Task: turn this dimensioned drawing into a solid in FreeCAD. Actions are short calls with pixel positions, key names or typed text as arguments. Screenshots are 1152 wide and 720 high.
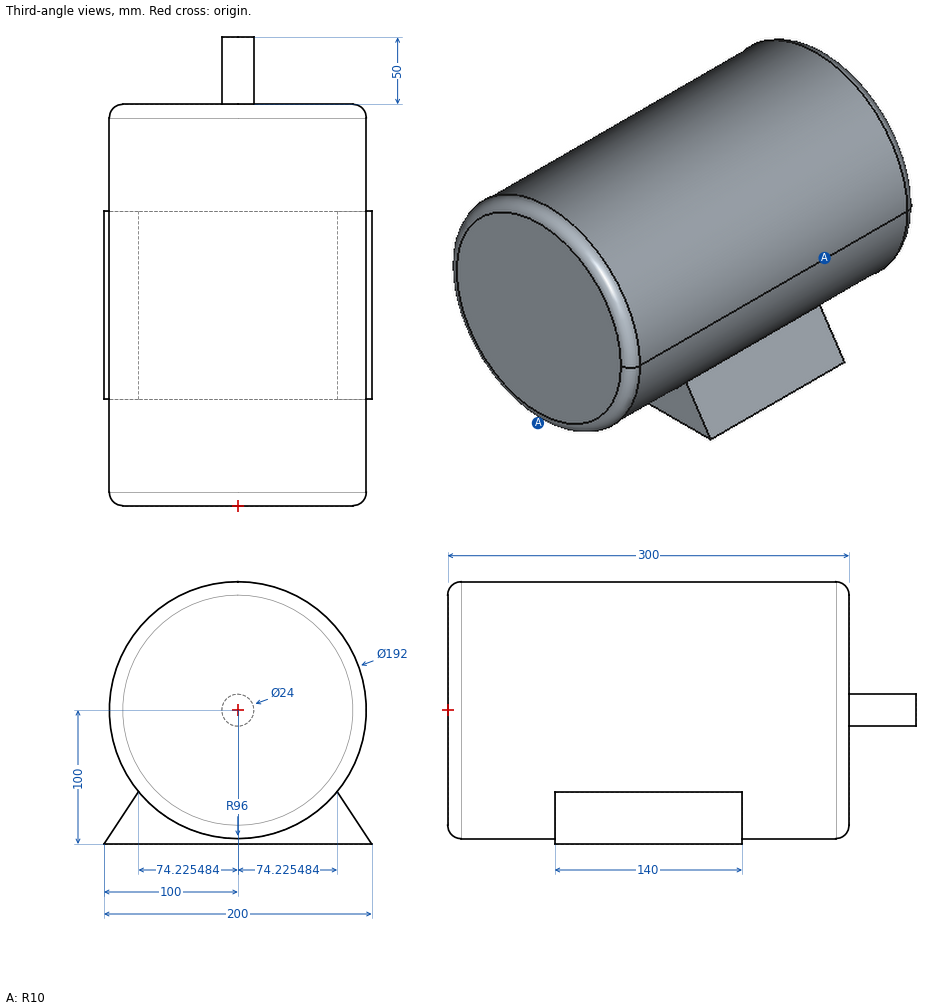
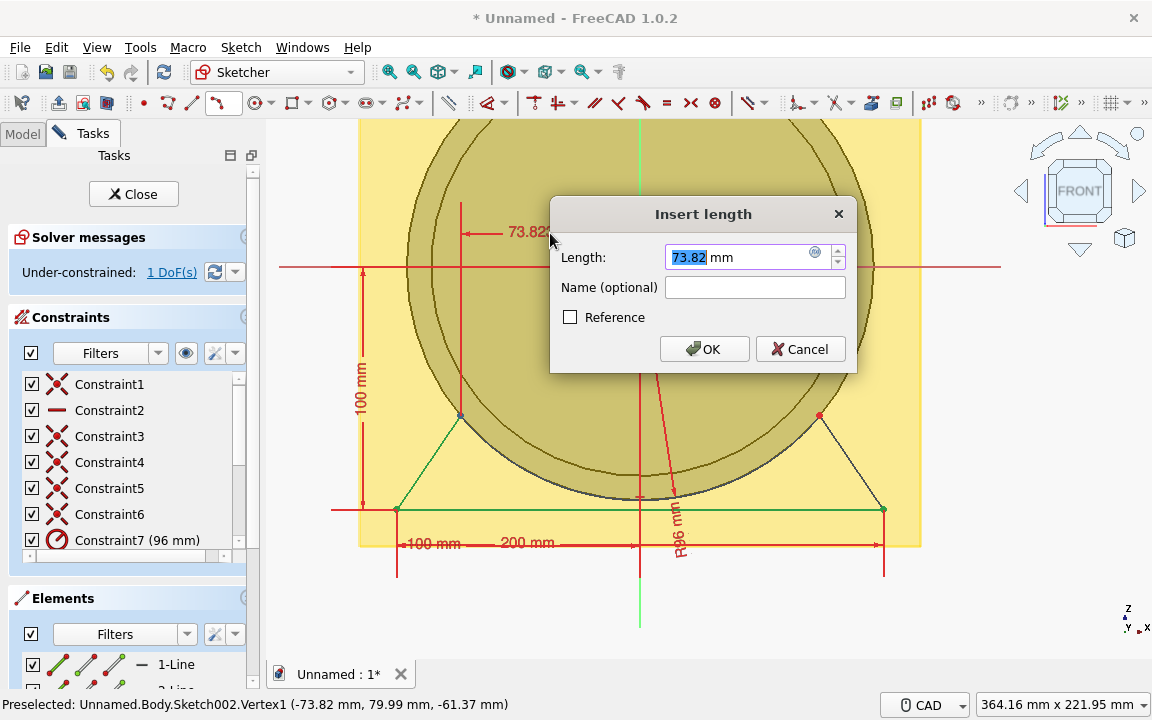
text(74.225484)
key(Return)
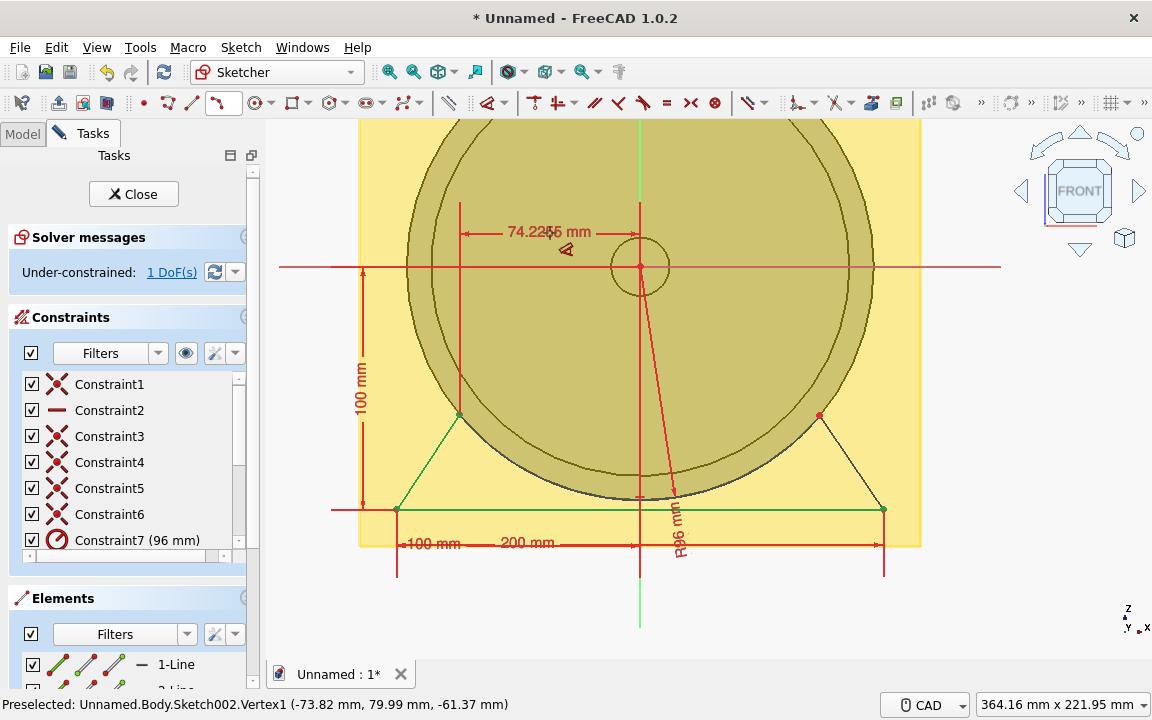
click(820, 416)
click(730, 233)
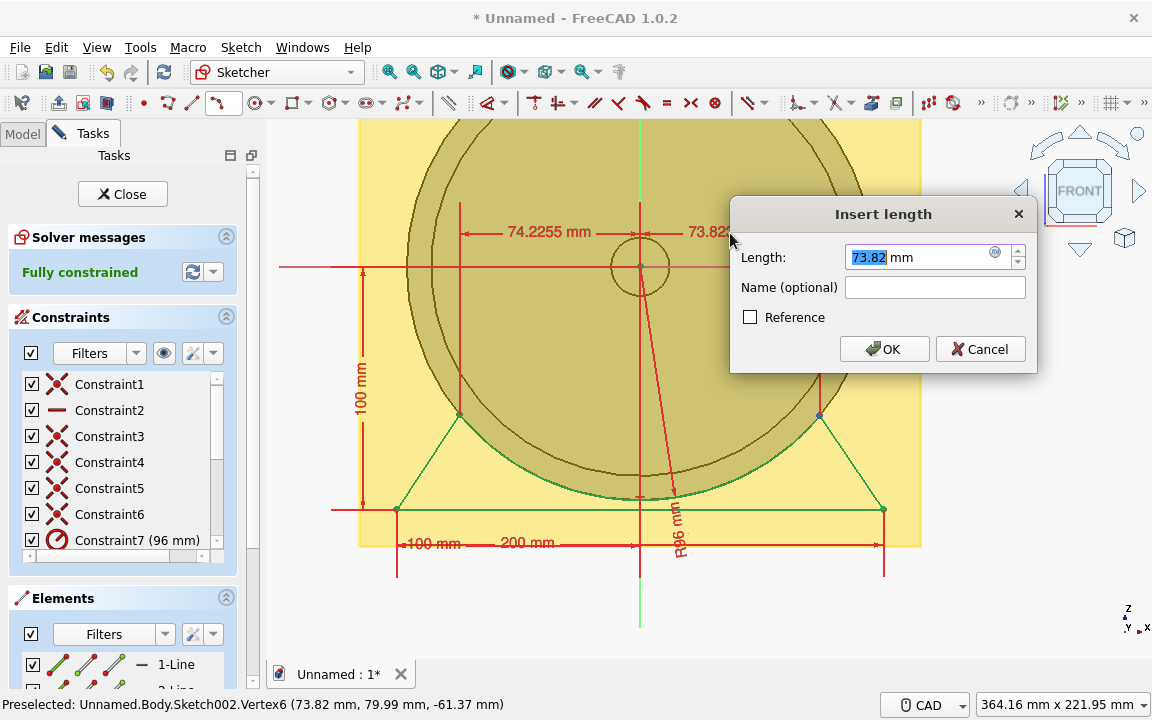
text(74.225484)
key(Return)
key(Escape)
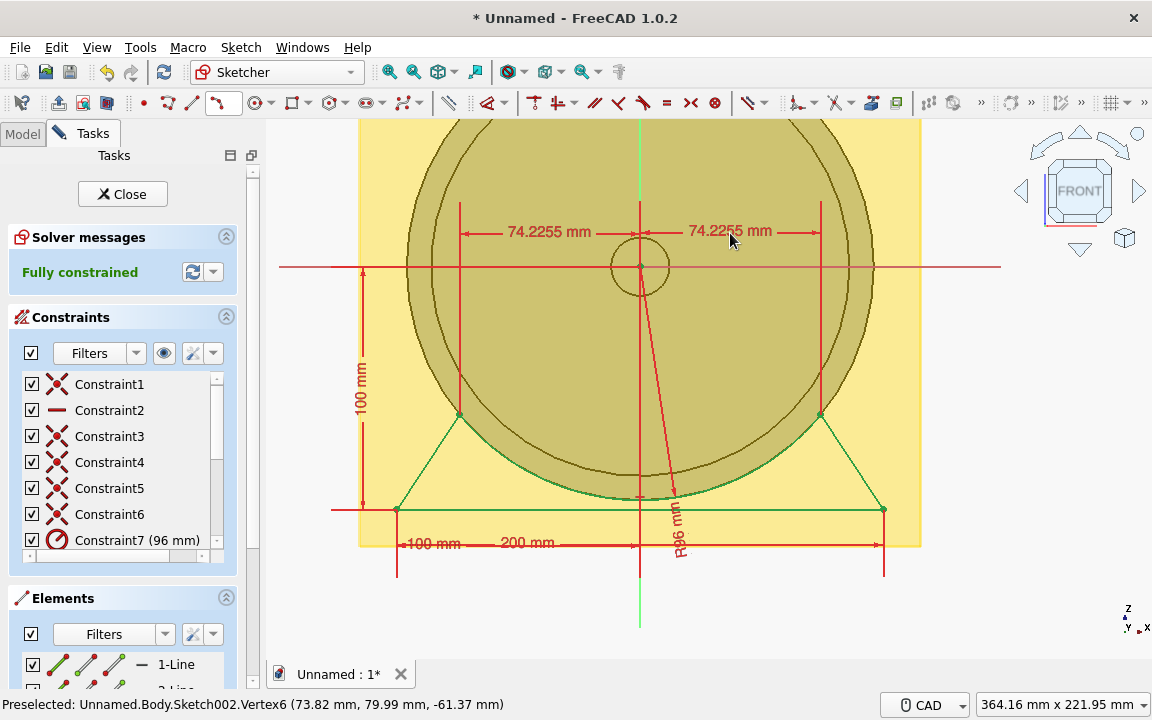
click(123, 194)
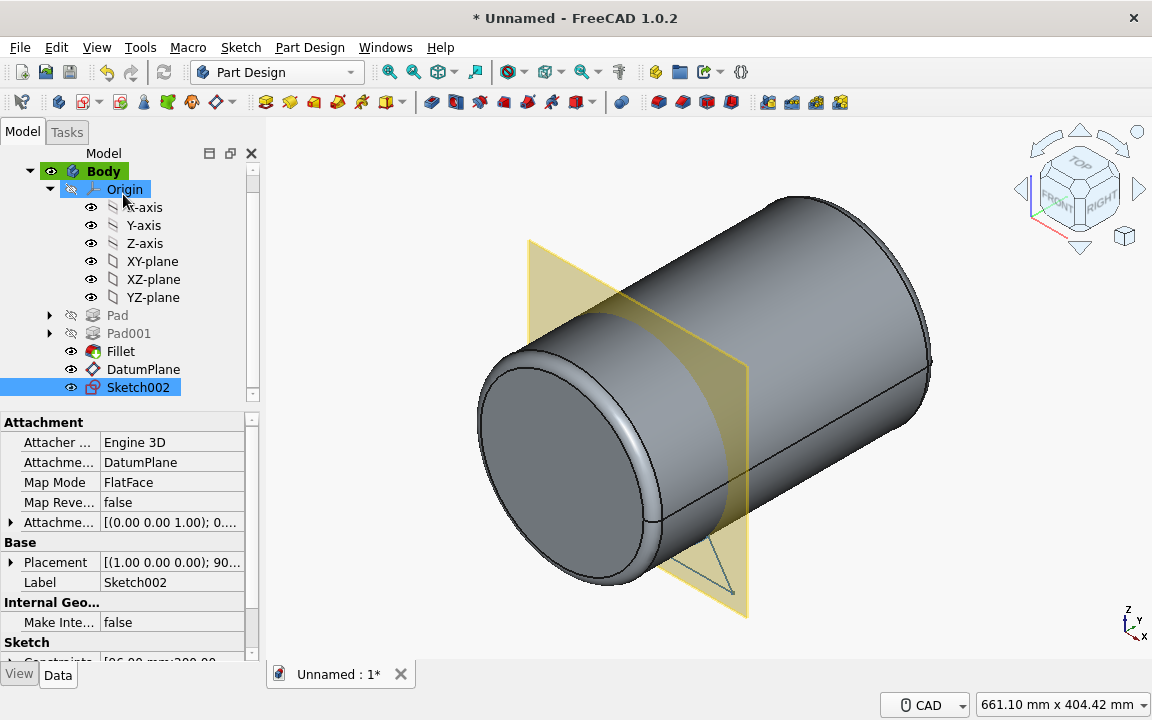
click(266, 102)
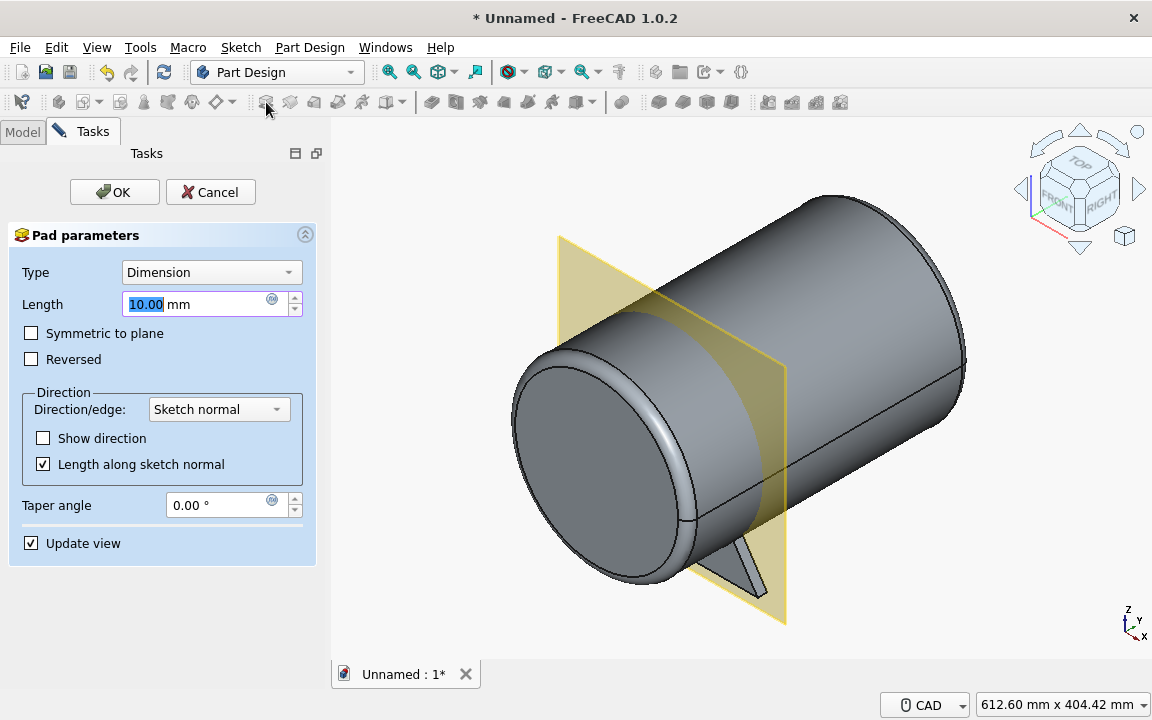
text(140)
key(Tab)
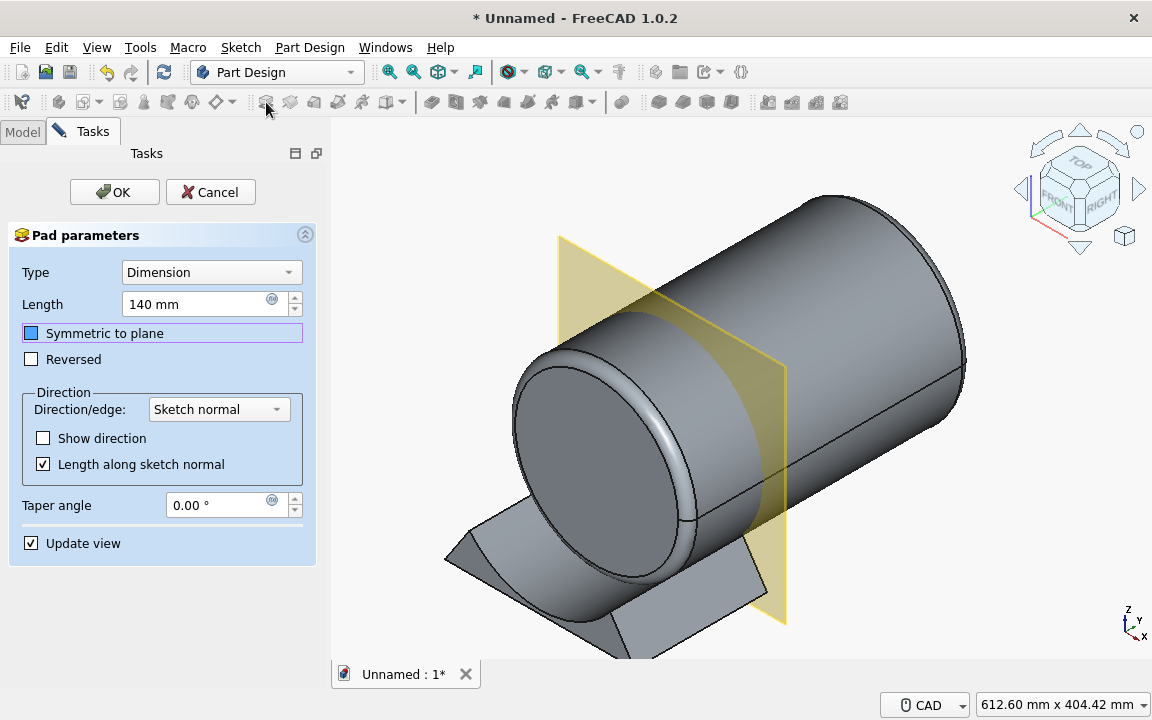
click(30, 359)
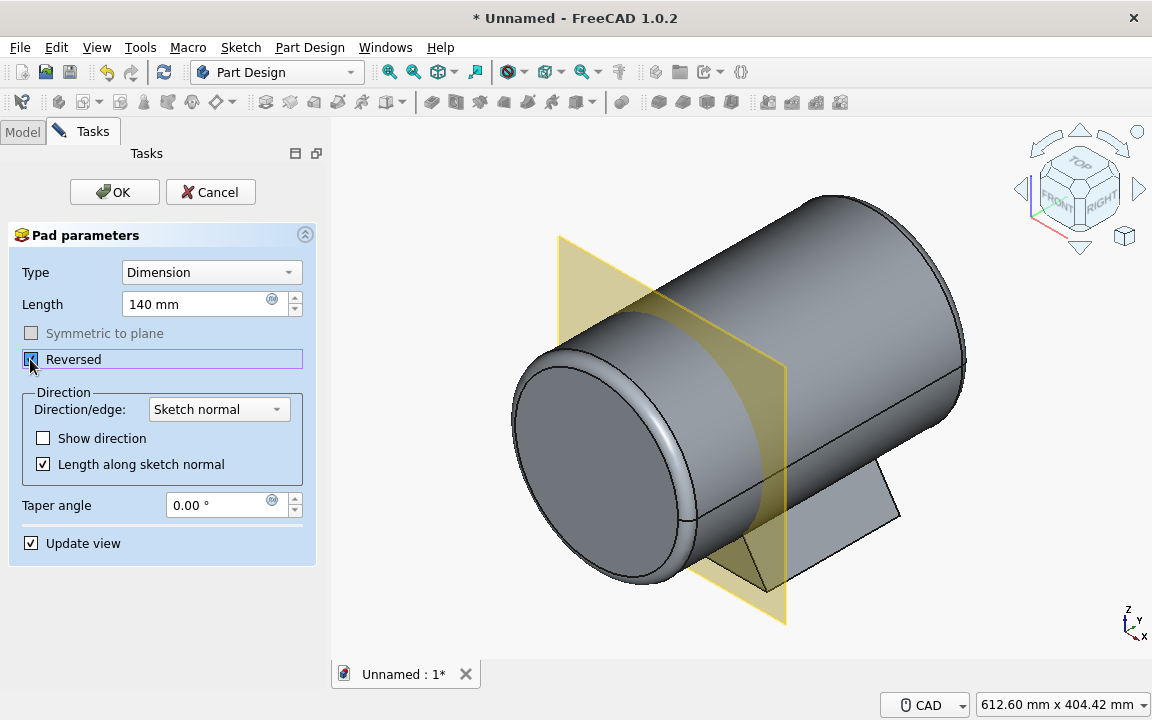
click(115, 192)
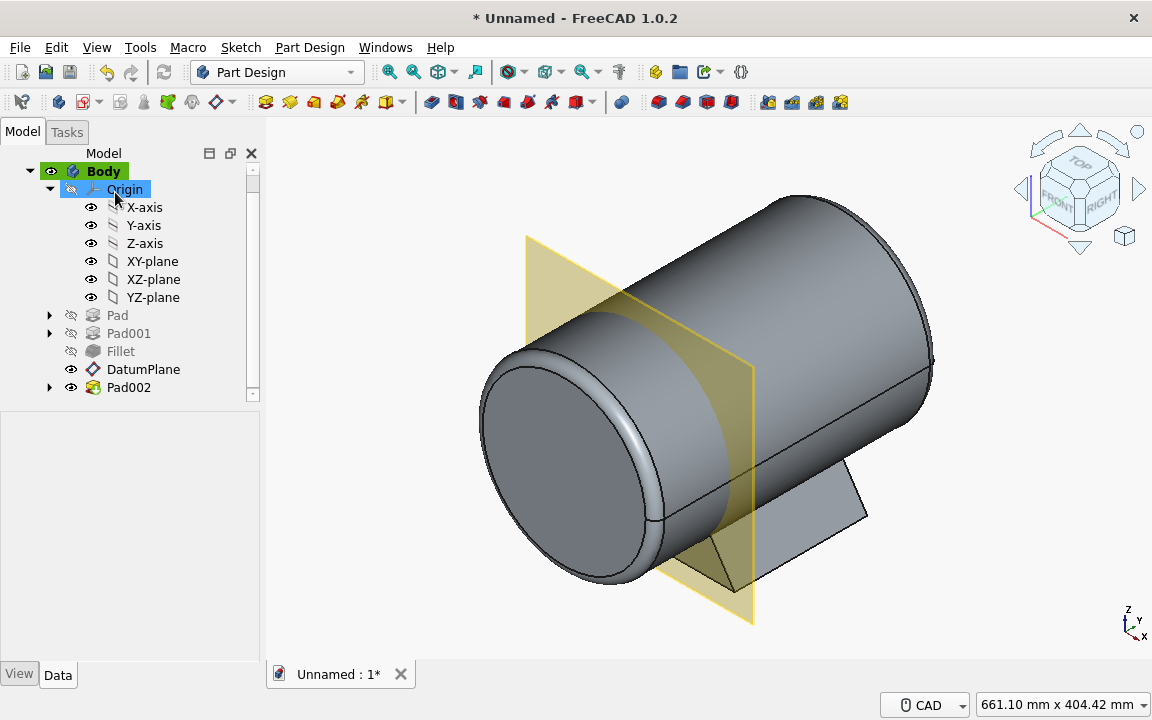
click(116, 369)
key(space)